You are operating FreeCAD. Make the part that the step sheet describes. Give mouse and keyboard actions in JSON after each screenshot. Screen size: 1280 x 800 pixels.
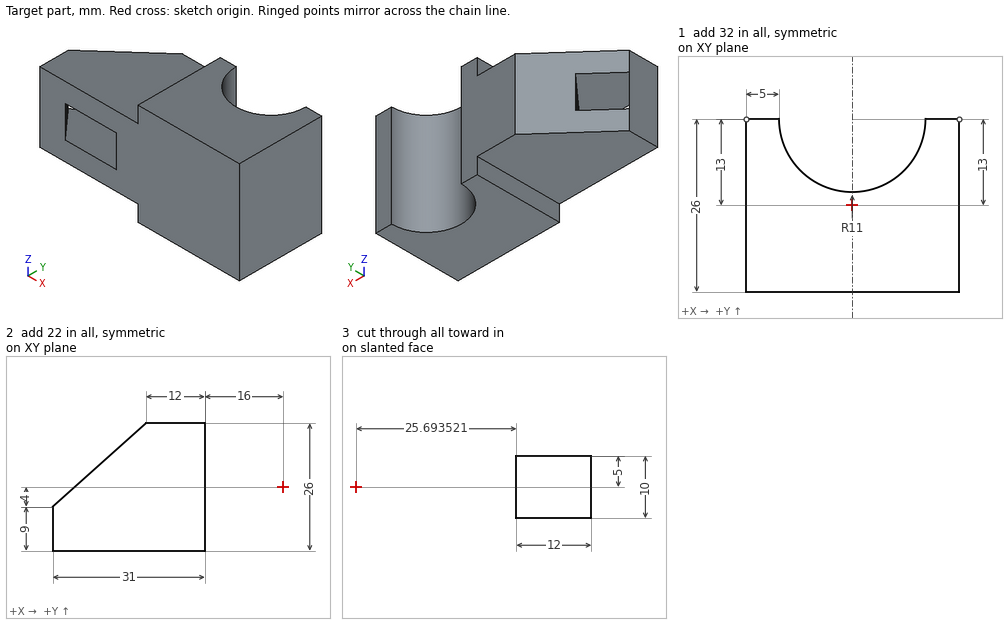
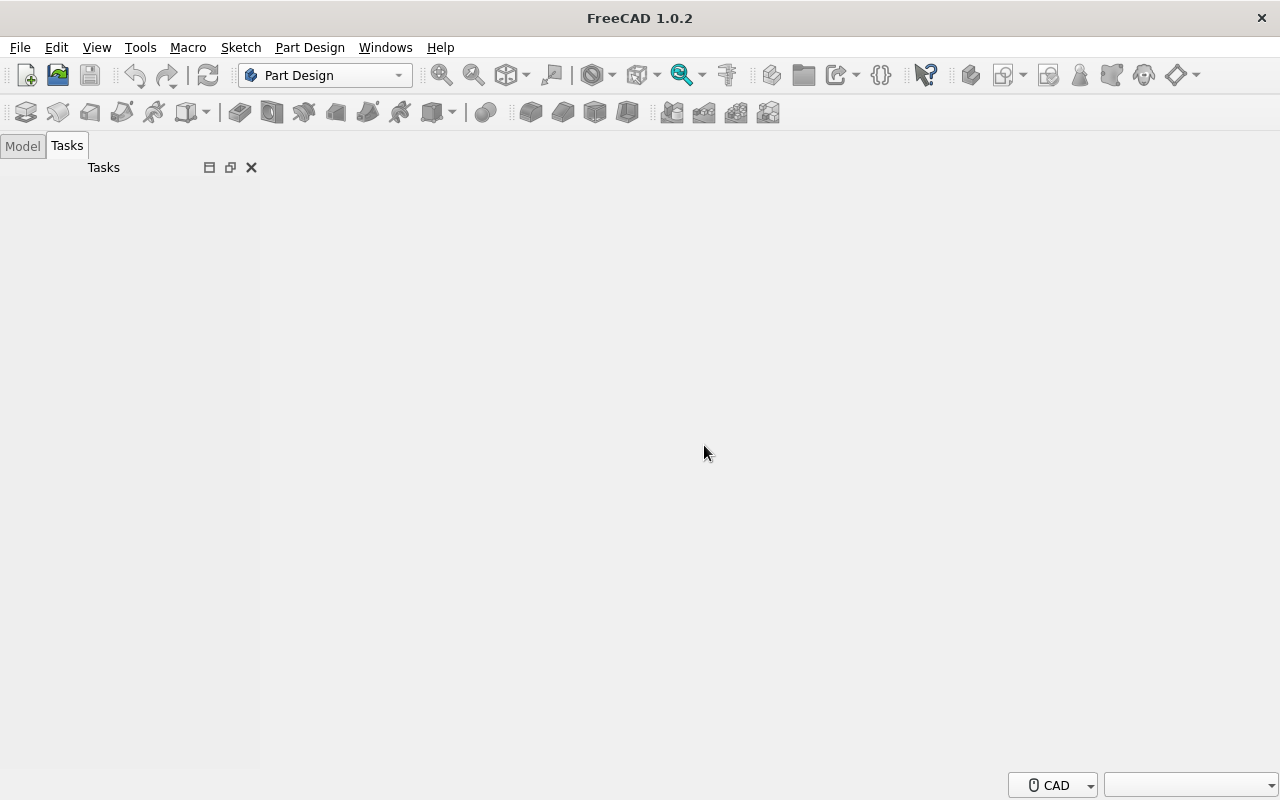
{"action": "key", "text": "ctrl+n"}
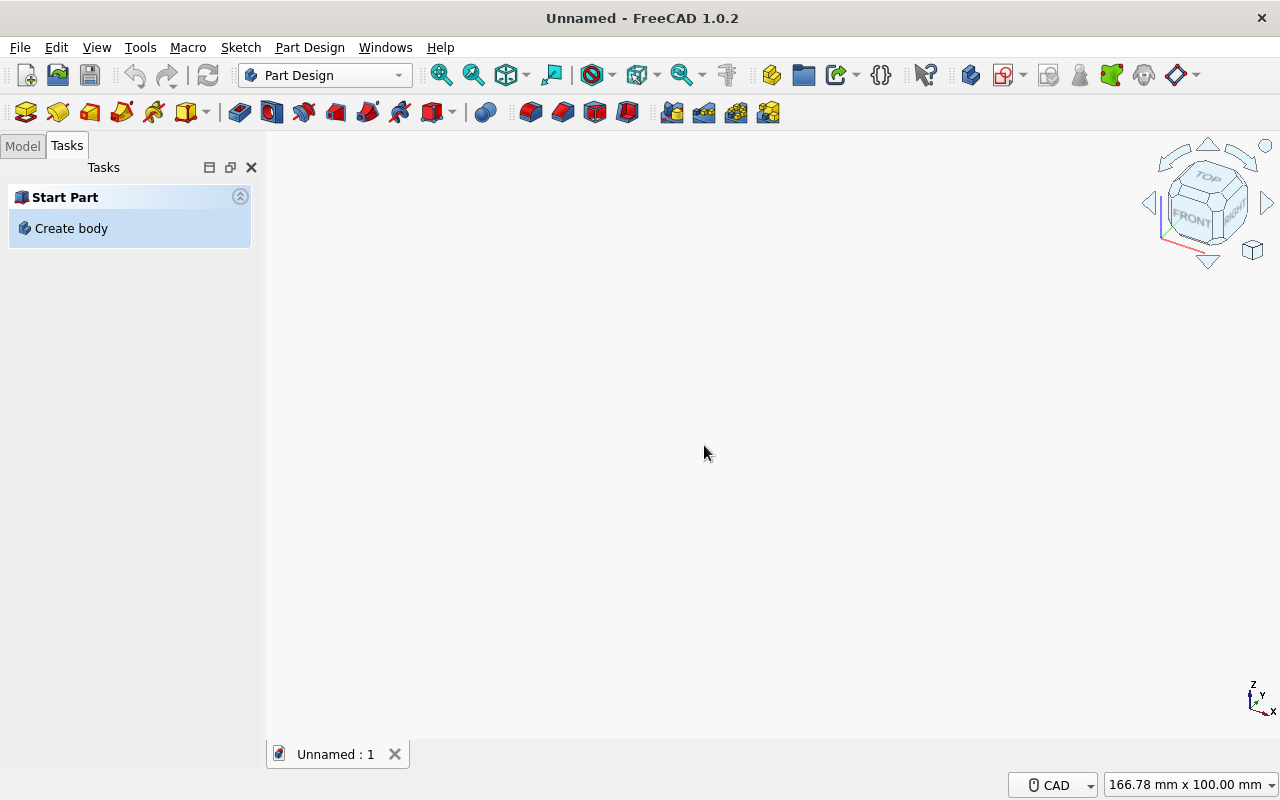
{"action": "left_click", "coordinate": [1004, 76]}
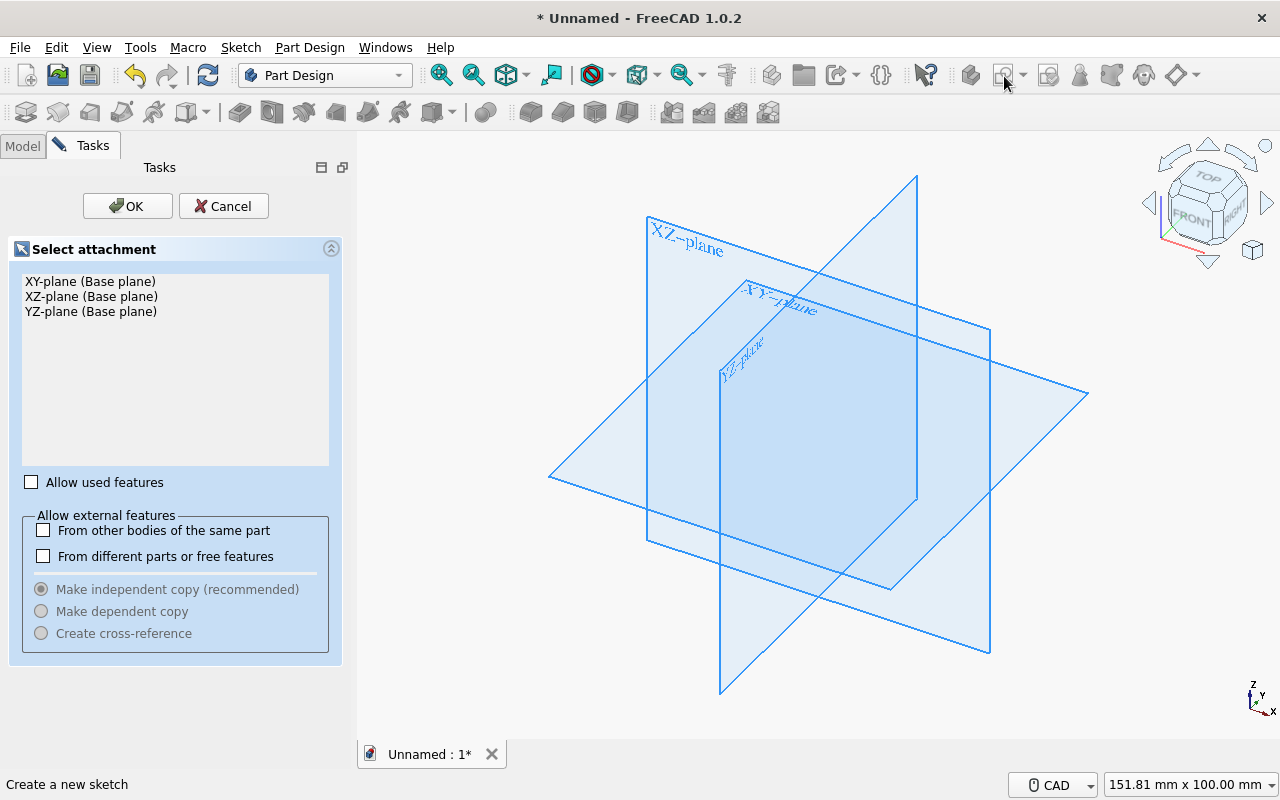
{"action": "left_click", "coordinate": [82, 282]}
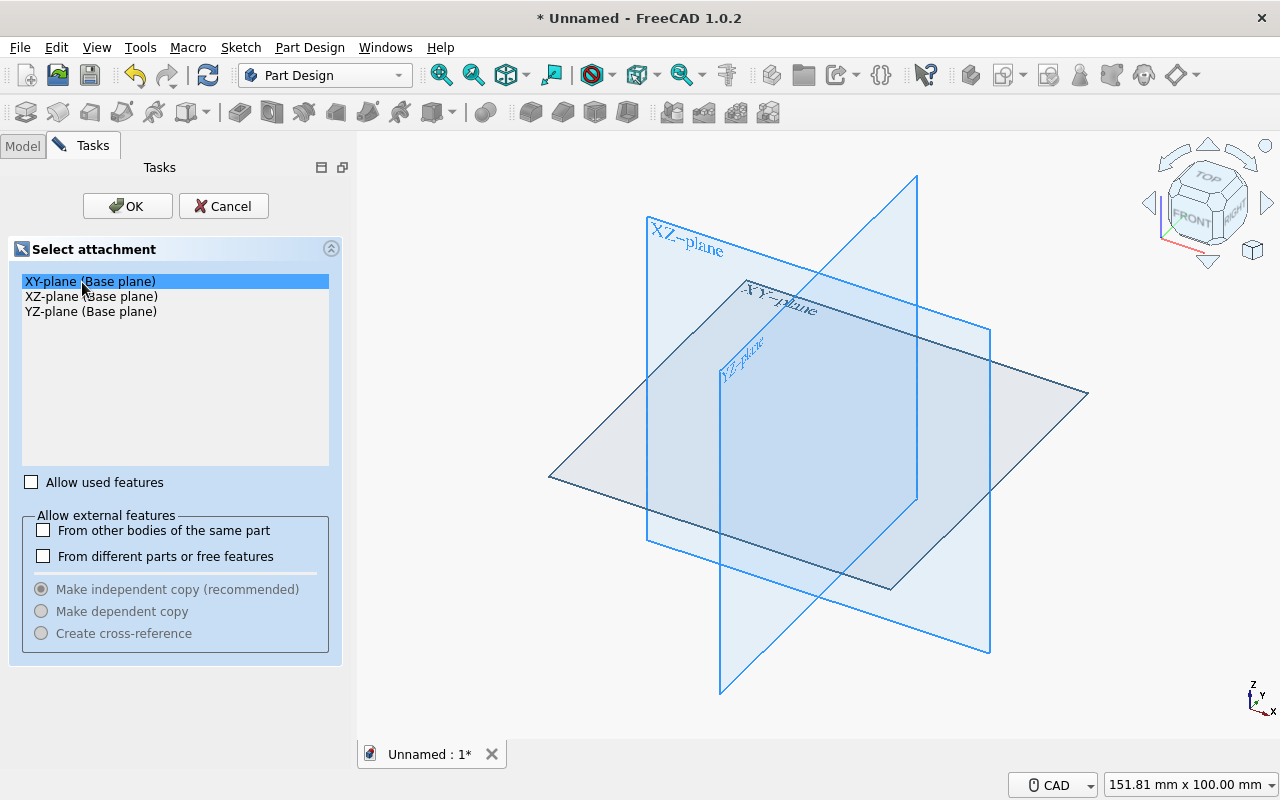
{"action": "left_click", "coordinate": [128, 206]}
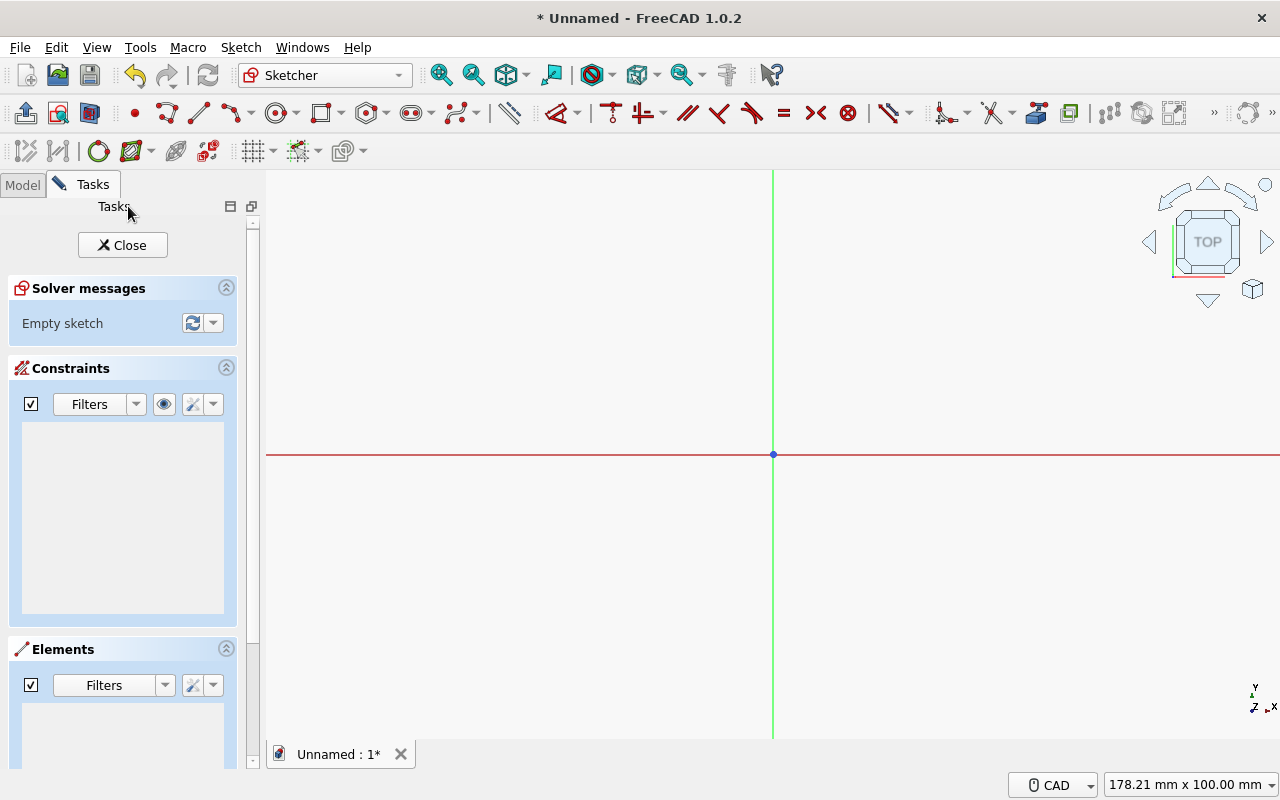
{"action": "scroll", "coordinate": [829, 455], "scroll_direction": "up", "scroll_amount": 4}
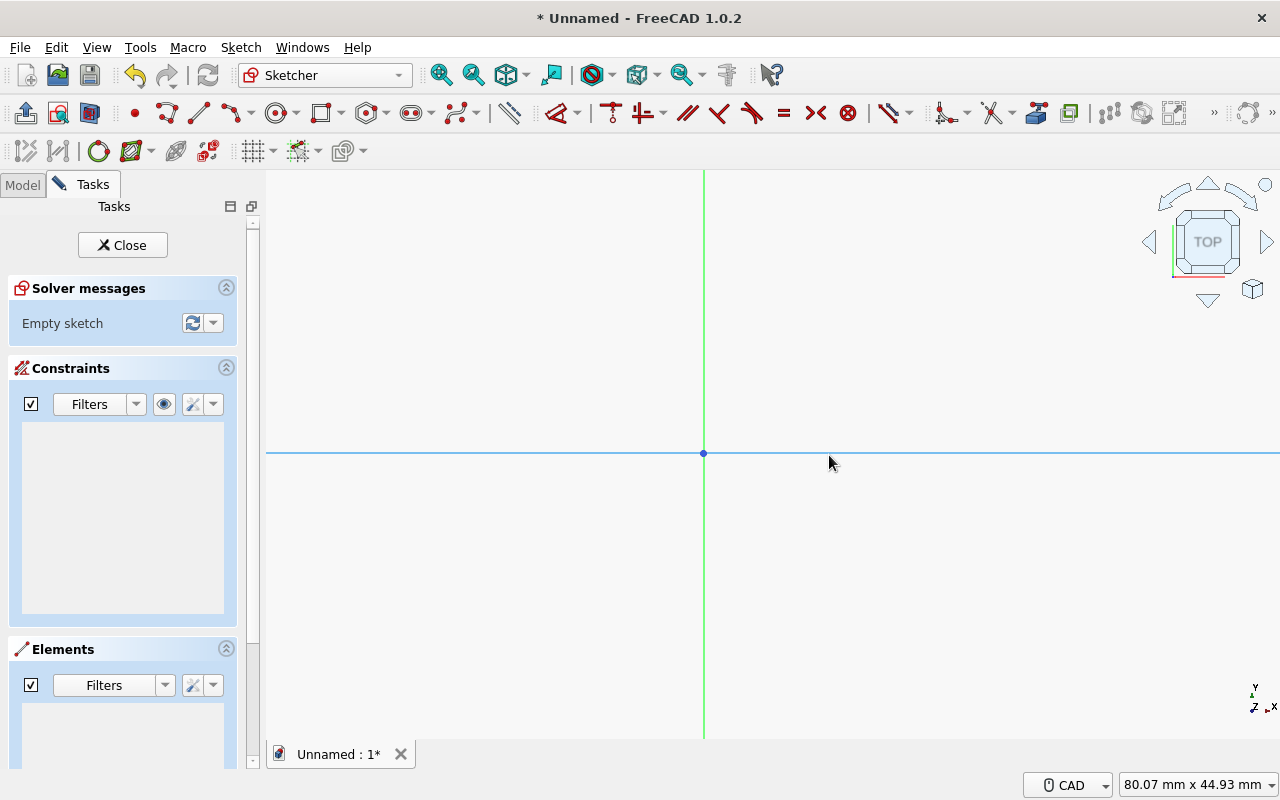
{"action": "left_click", "coordinate": [168, 114]}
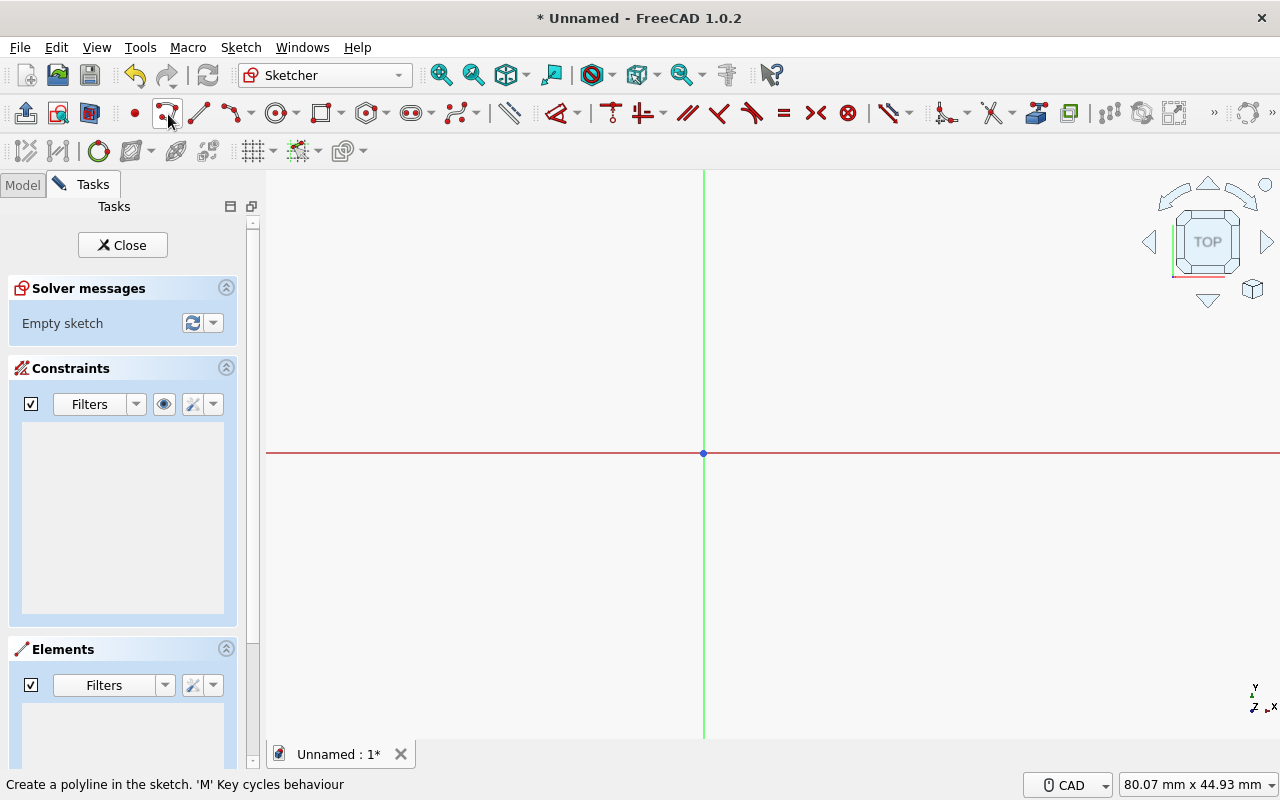
{"action": "left_click", "coordinate": [564, 289]}
{"action": "left_click", "coordinate": [501, 289]}
{"action": "left_click", "coordinate": [501, 618]}
{"action": "left_click", "coordinate": [906, 618]}
{"action": "left_click", "coordinate": [906, 289]}
{"action": "left_click", "coordinate": [843, 289]}
{"action": "right_click", "coordinate": [843, 289]}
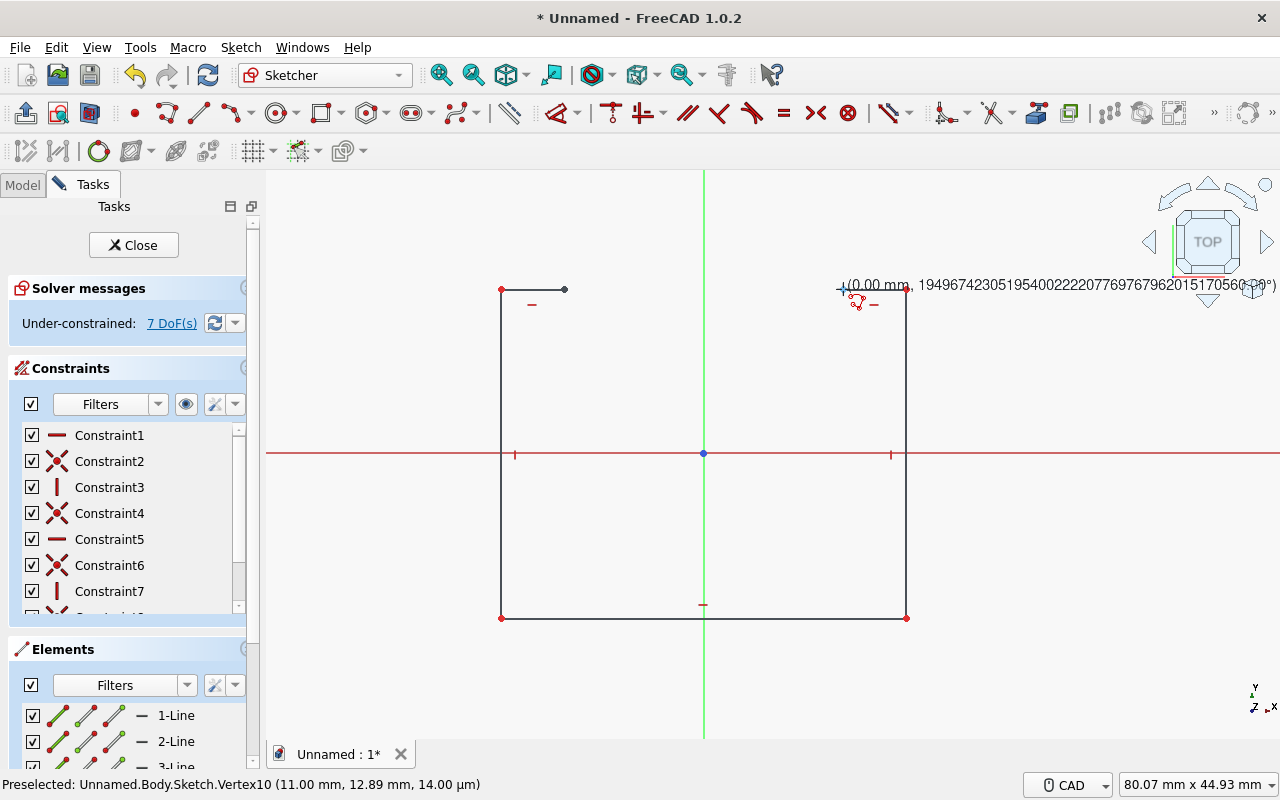
{"action": "key", "text": "g 3 a"}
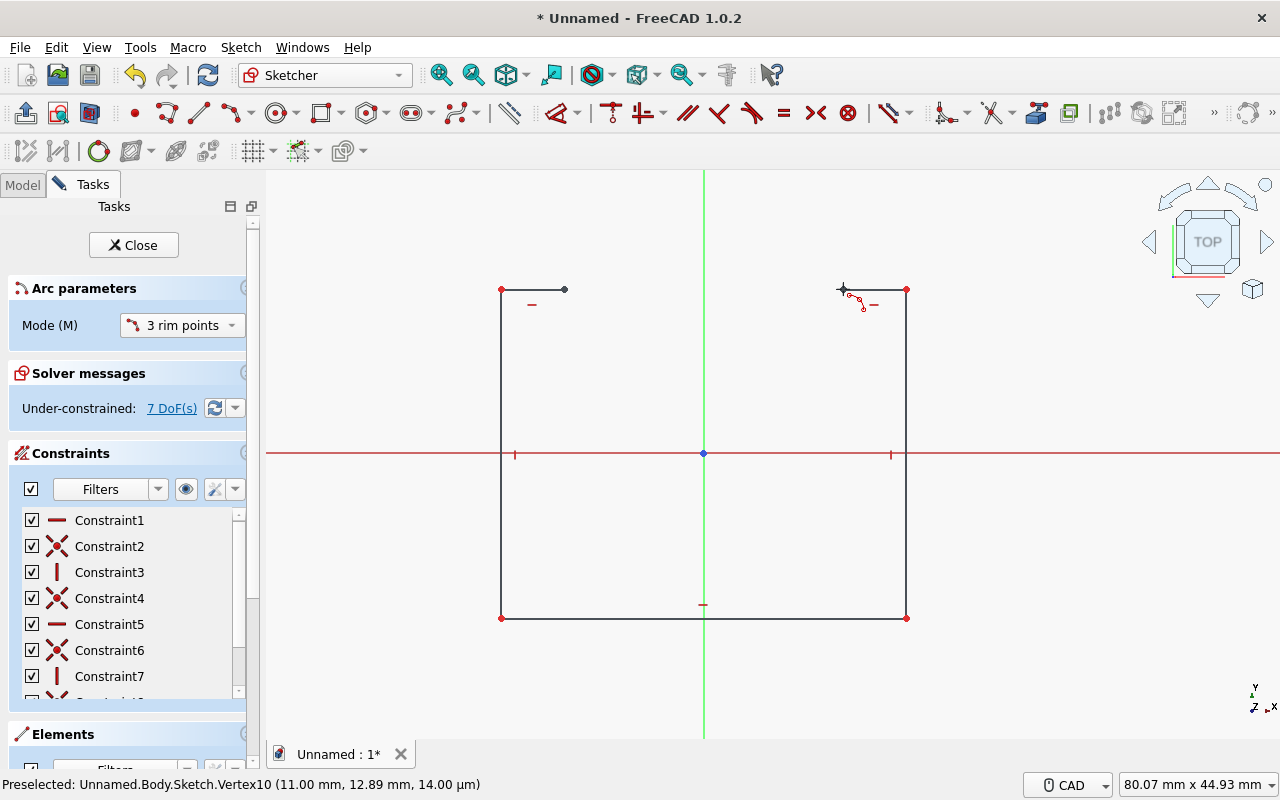
{"action": "left_click", "coordinate": [843, 290]}
{"action": "left_click", "coordinate": [564, 290]}
{"action": "left_click", "coordinate": [661, 421]}
{"action": "key", "text": "Escape"}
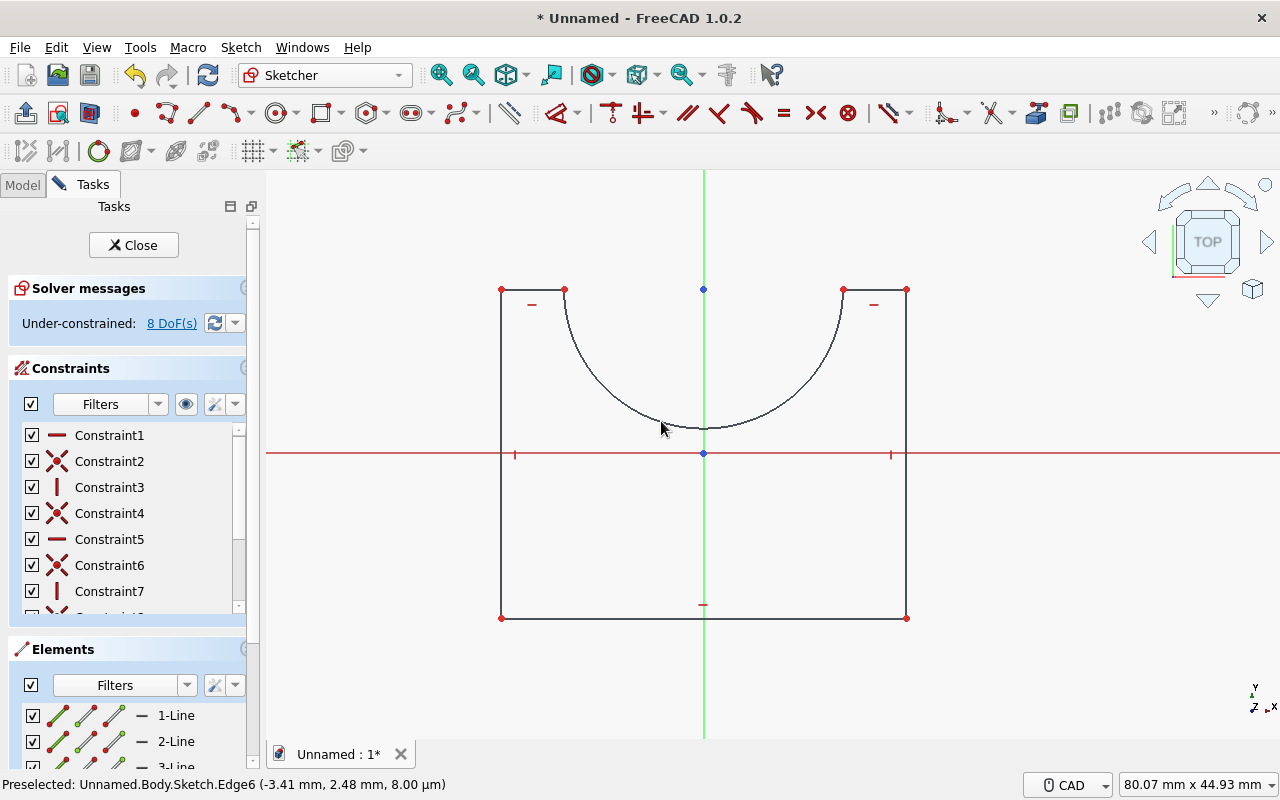
{"action": "left_click", "coordinate": [703, 289]}